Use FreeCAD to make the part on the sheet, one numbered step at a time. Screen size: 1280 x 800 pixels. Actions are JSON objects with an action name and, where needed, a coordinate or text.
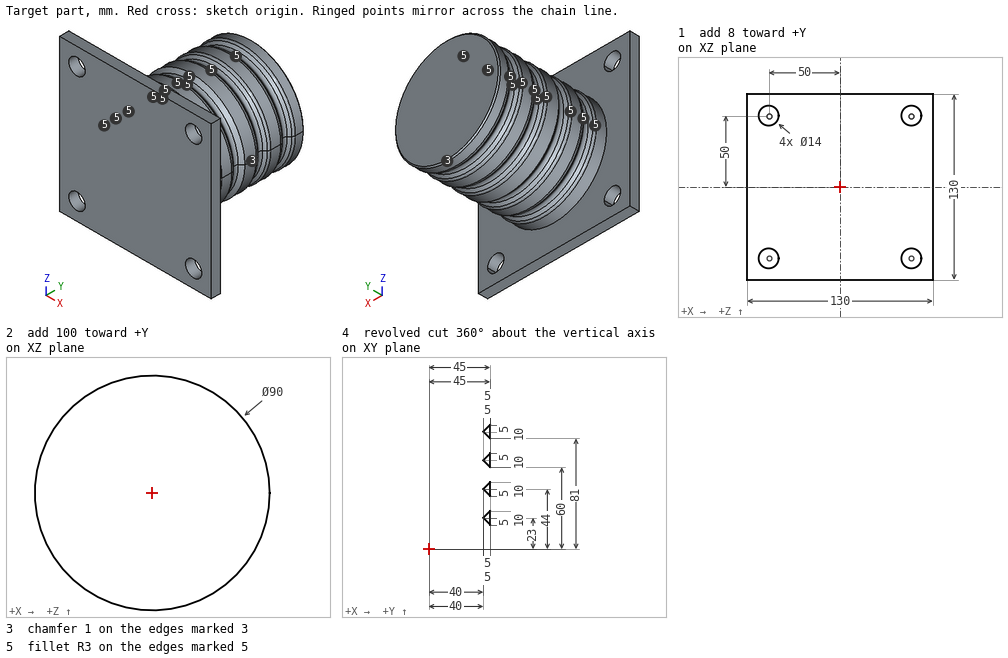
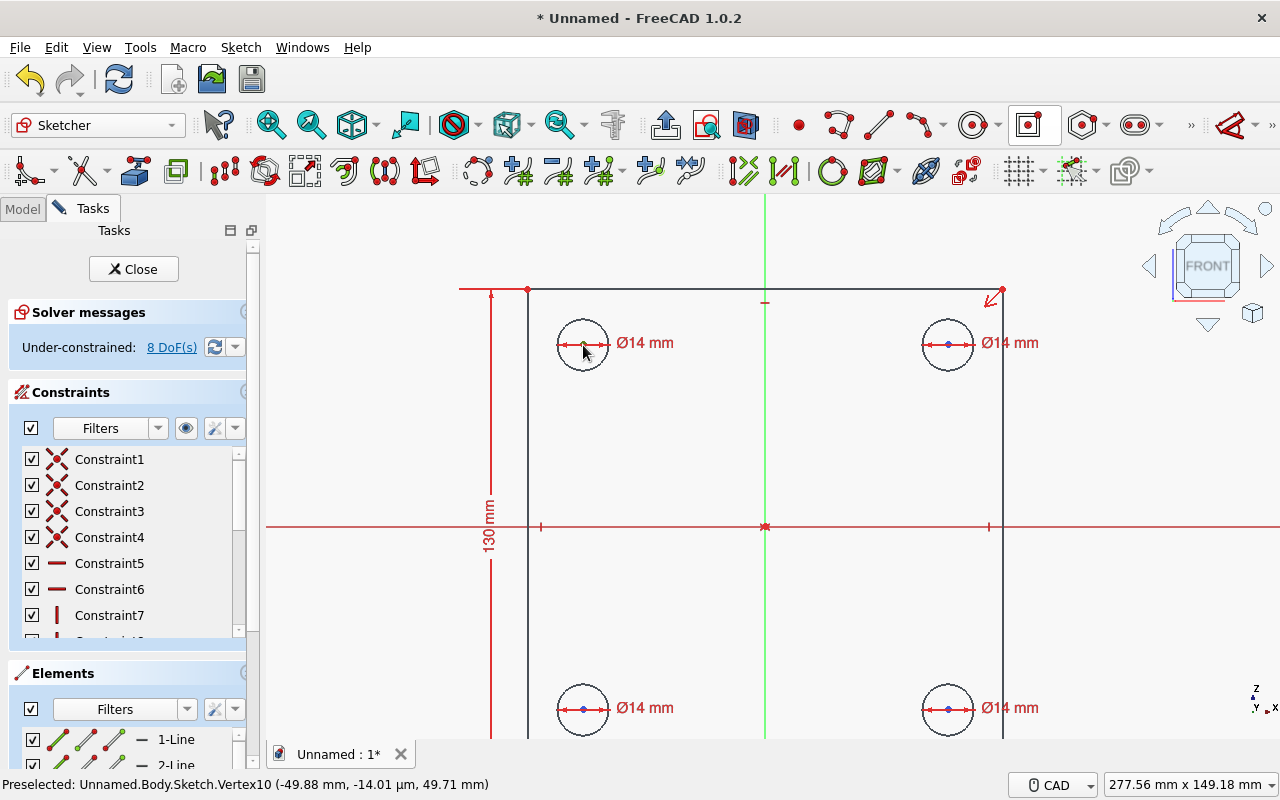
{"action": "left_click", "coordinate": [948, 345]}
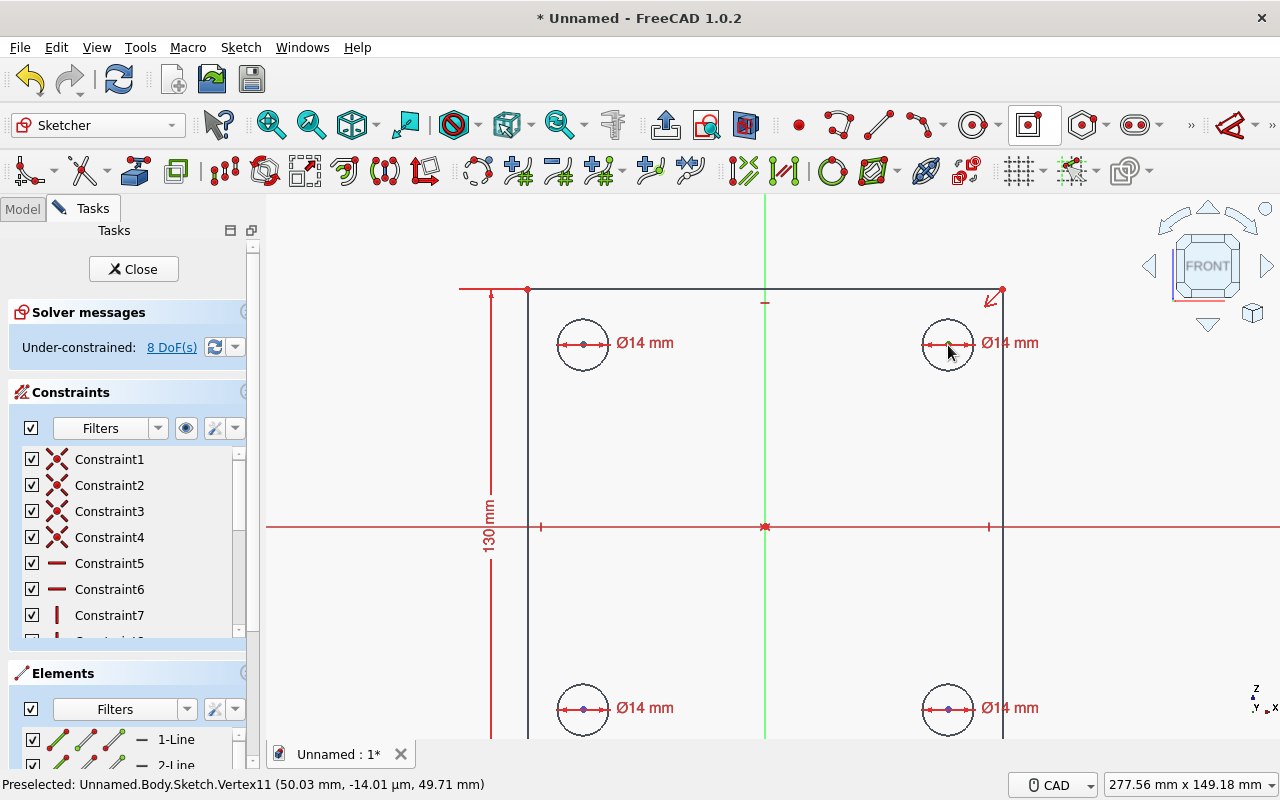
{"action": "left_click", "coordinate": [765, 676]}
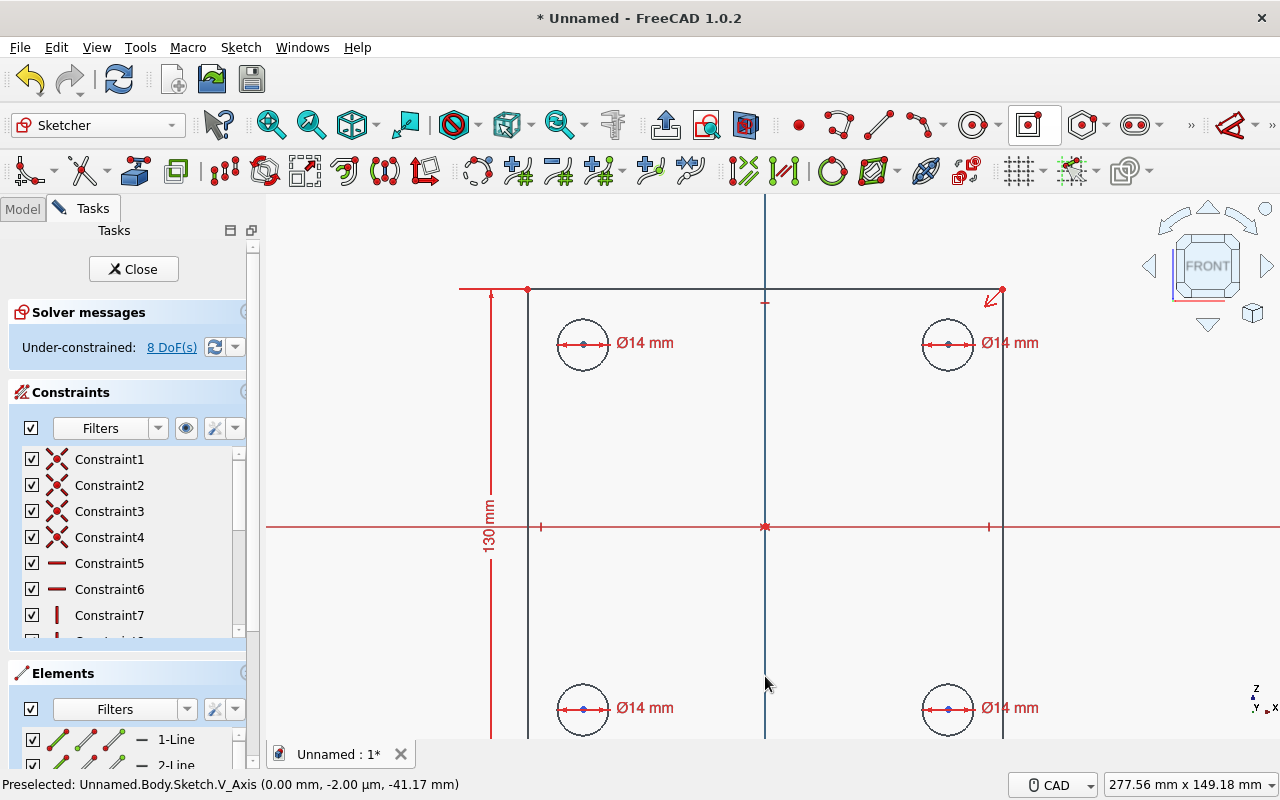
{"action": "key", "text": "s"}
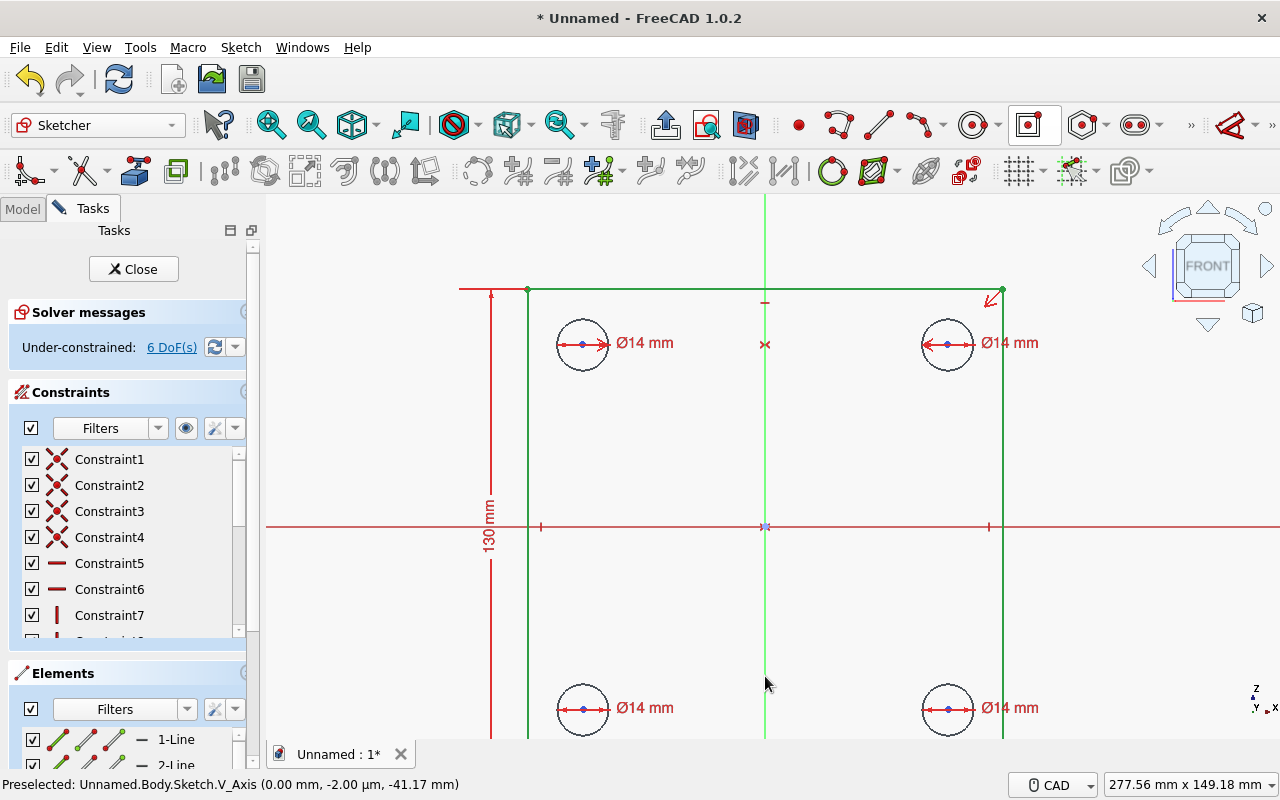
{"action": "left_click", "coordinate": [583, 345]}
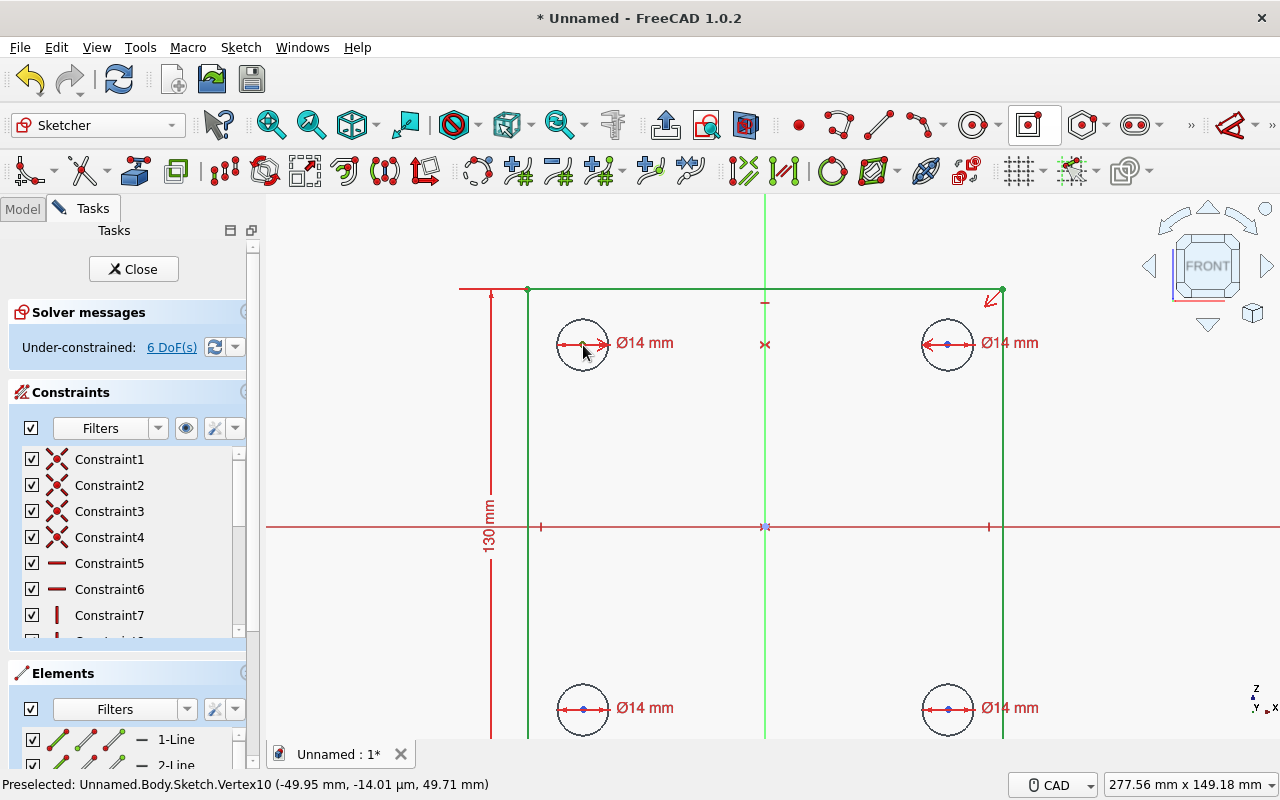
{"action": "left_click", "coordinate": [583, 710]}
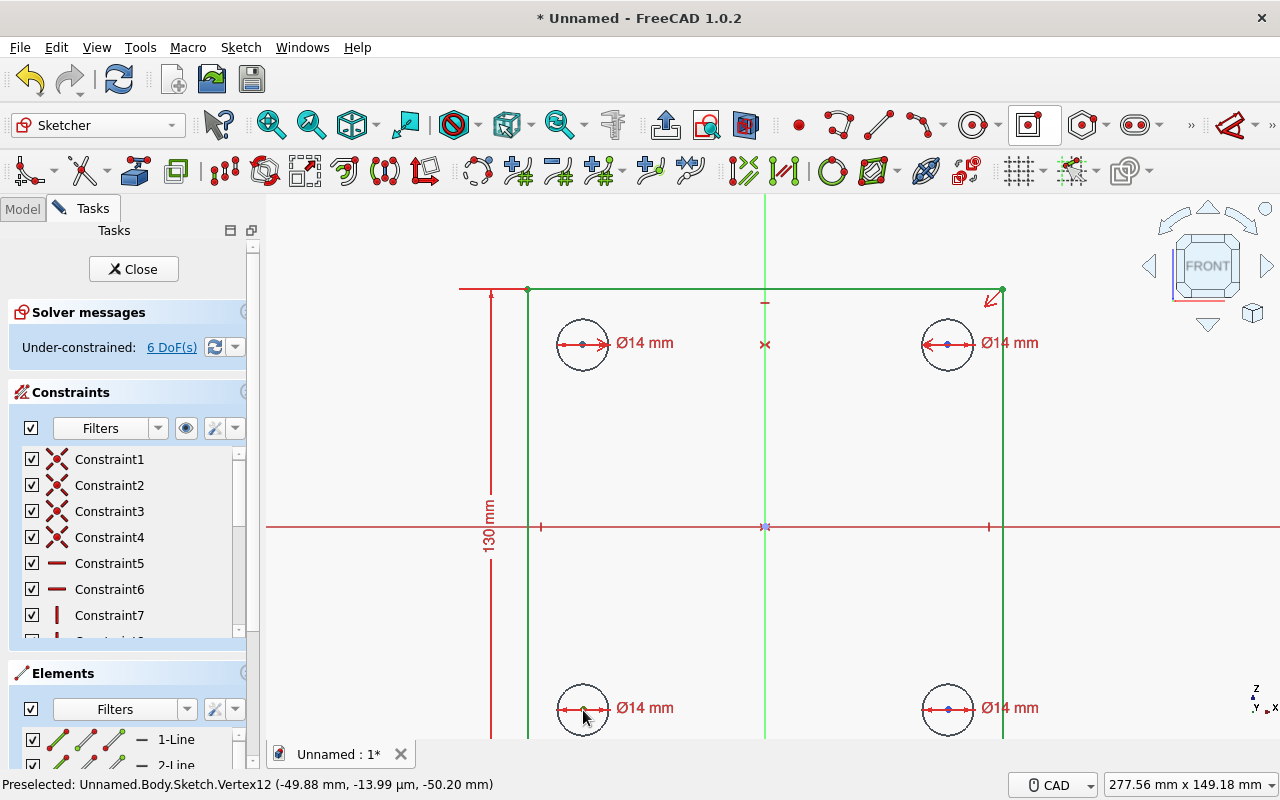
{"action": "left_click", "coordinate": [353, 527]}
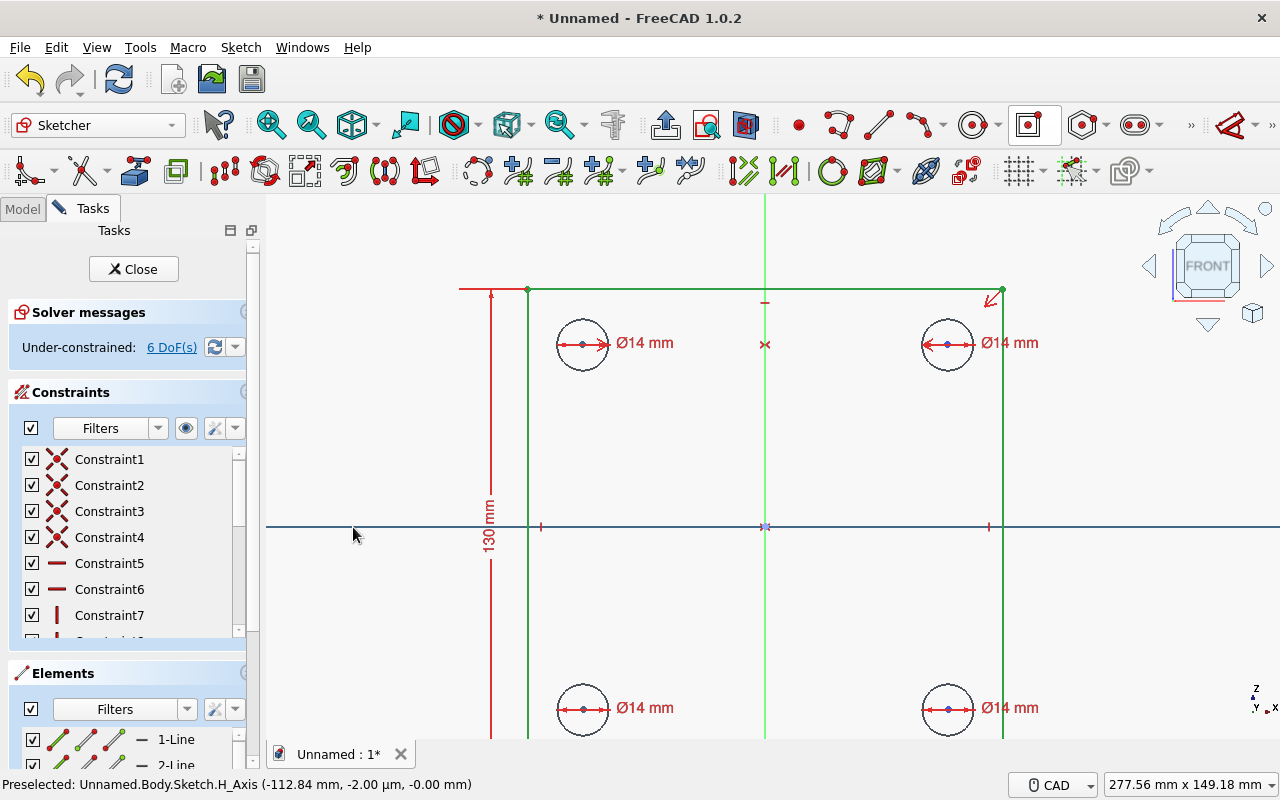
{"action": "key", "text": "s"}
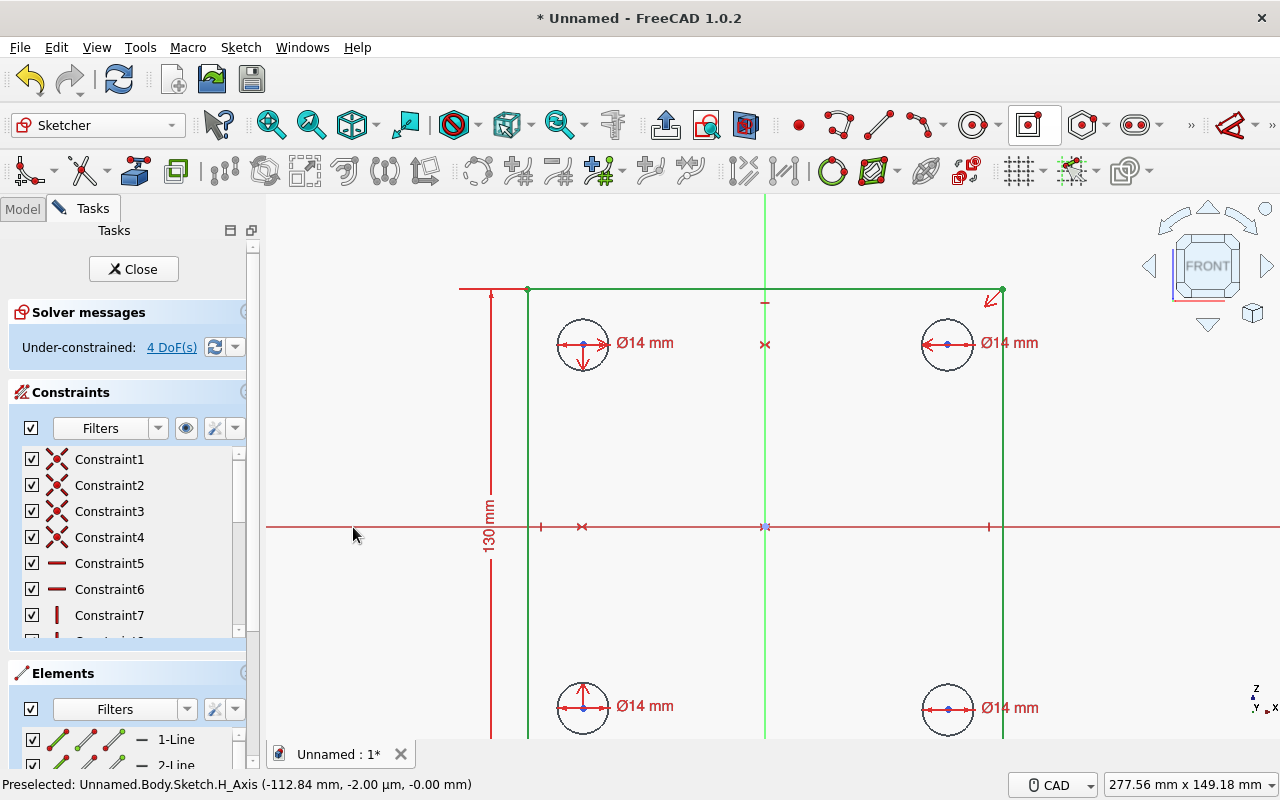
{"action": "left_click", "coordinate": [947, 345]}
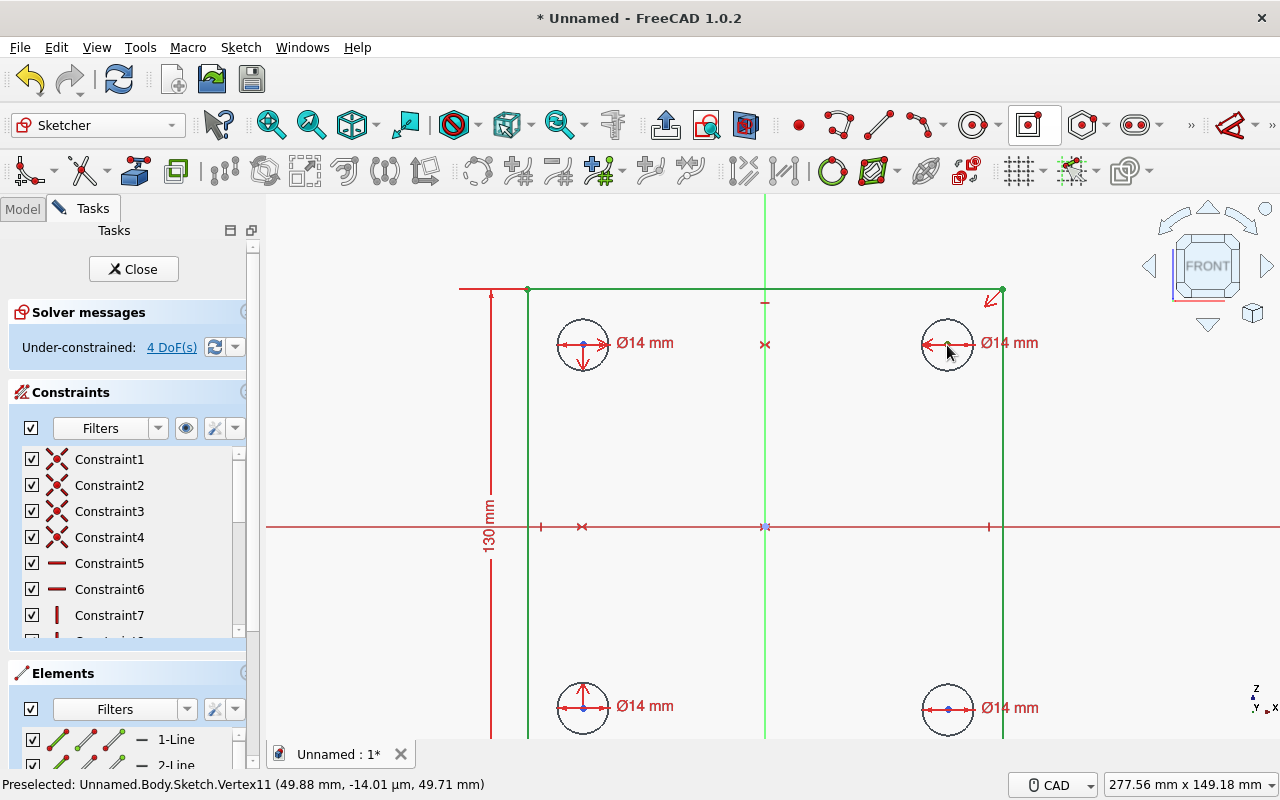
{"action": "left_click", "coordinate": [948, 710]}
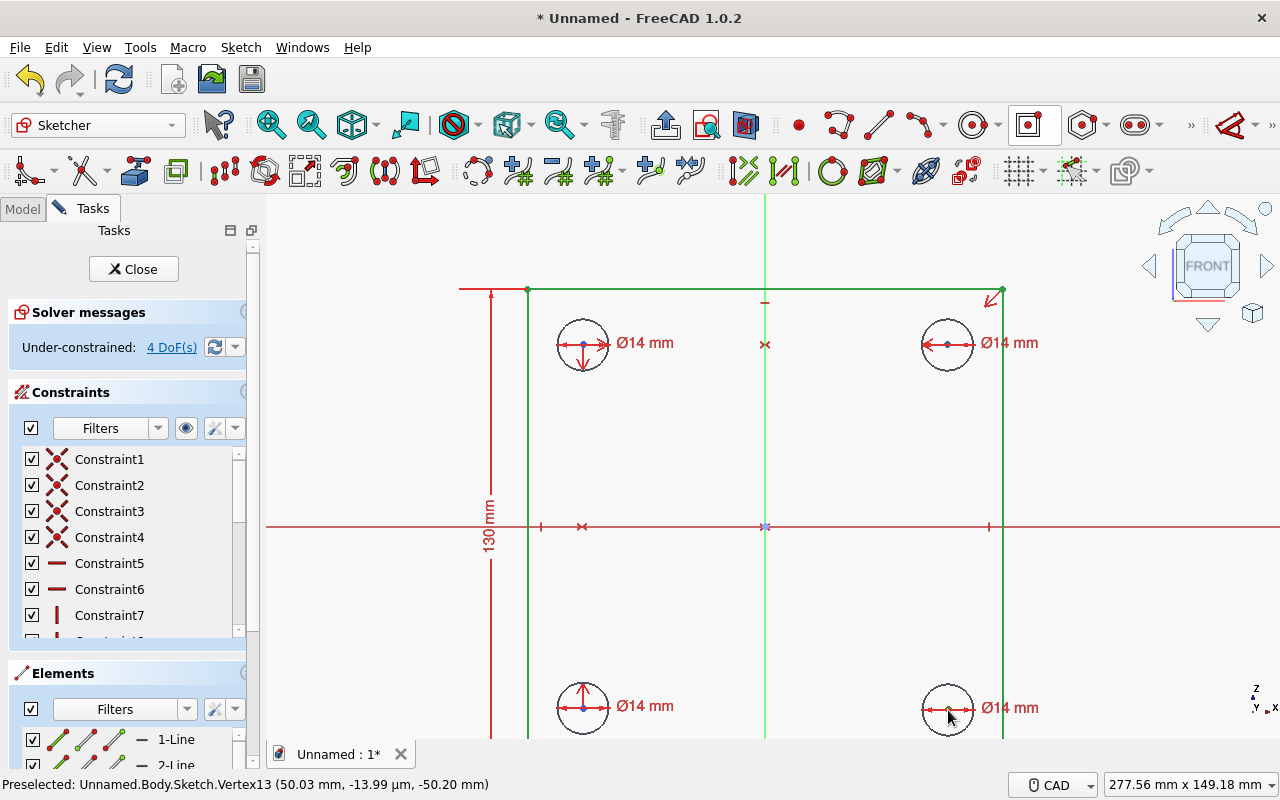
{"action": "left_click", "coordinate": [353, 527]}